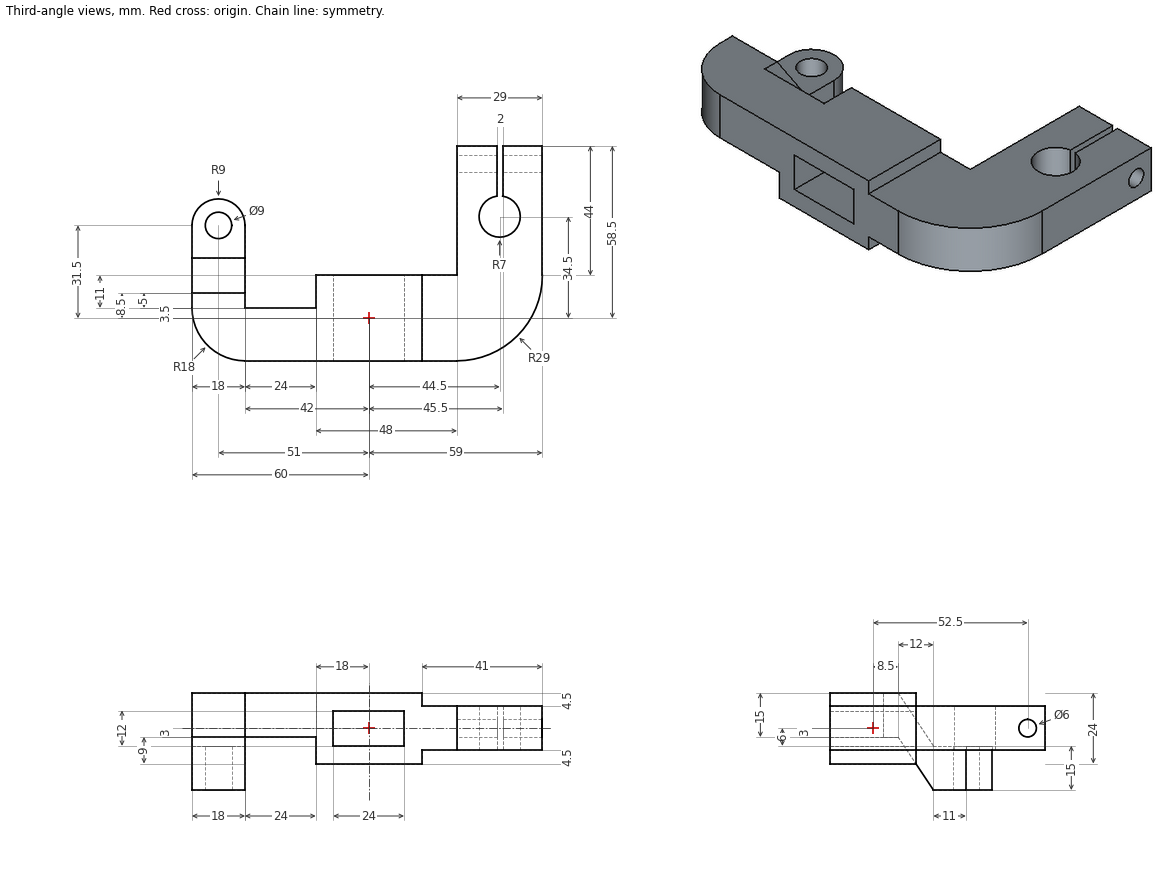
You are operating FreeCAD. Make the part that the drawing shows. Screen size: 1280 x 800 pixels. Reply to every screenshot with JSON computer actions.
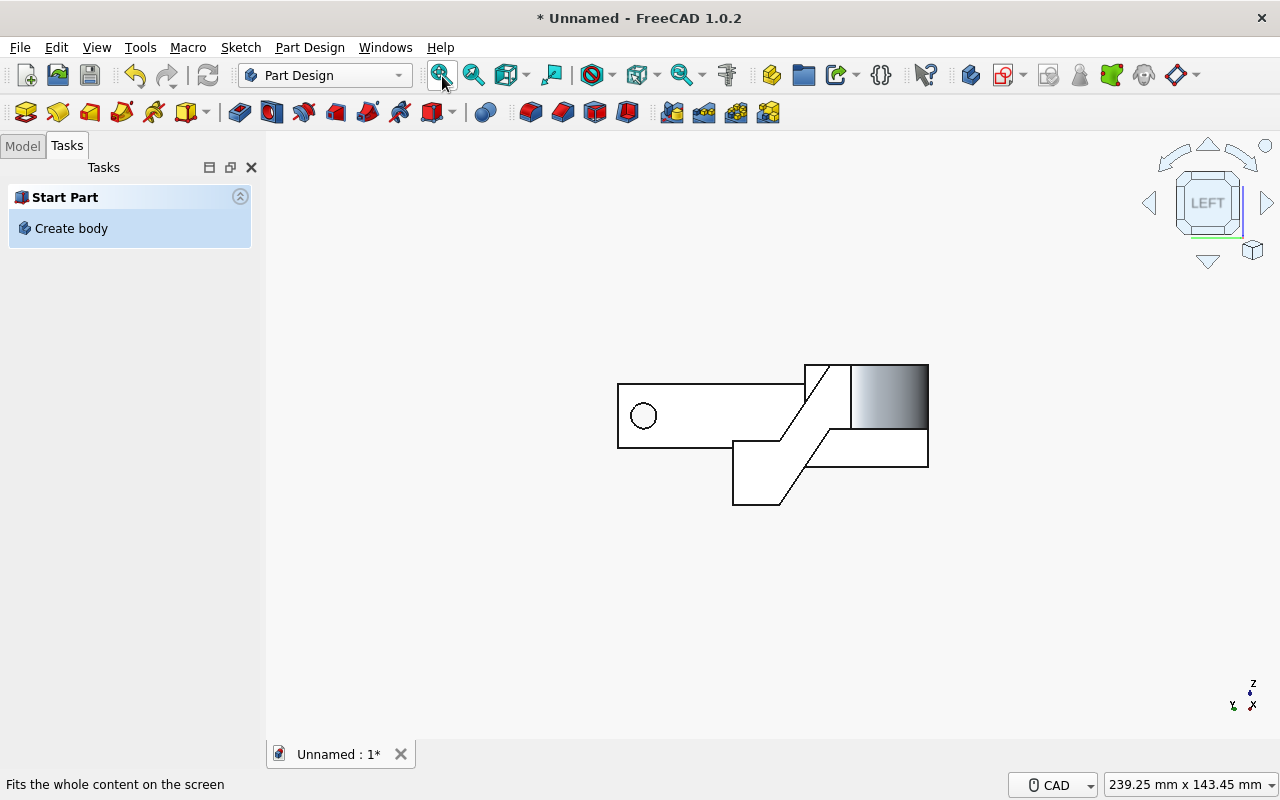
{"action": "key", "text": "0"}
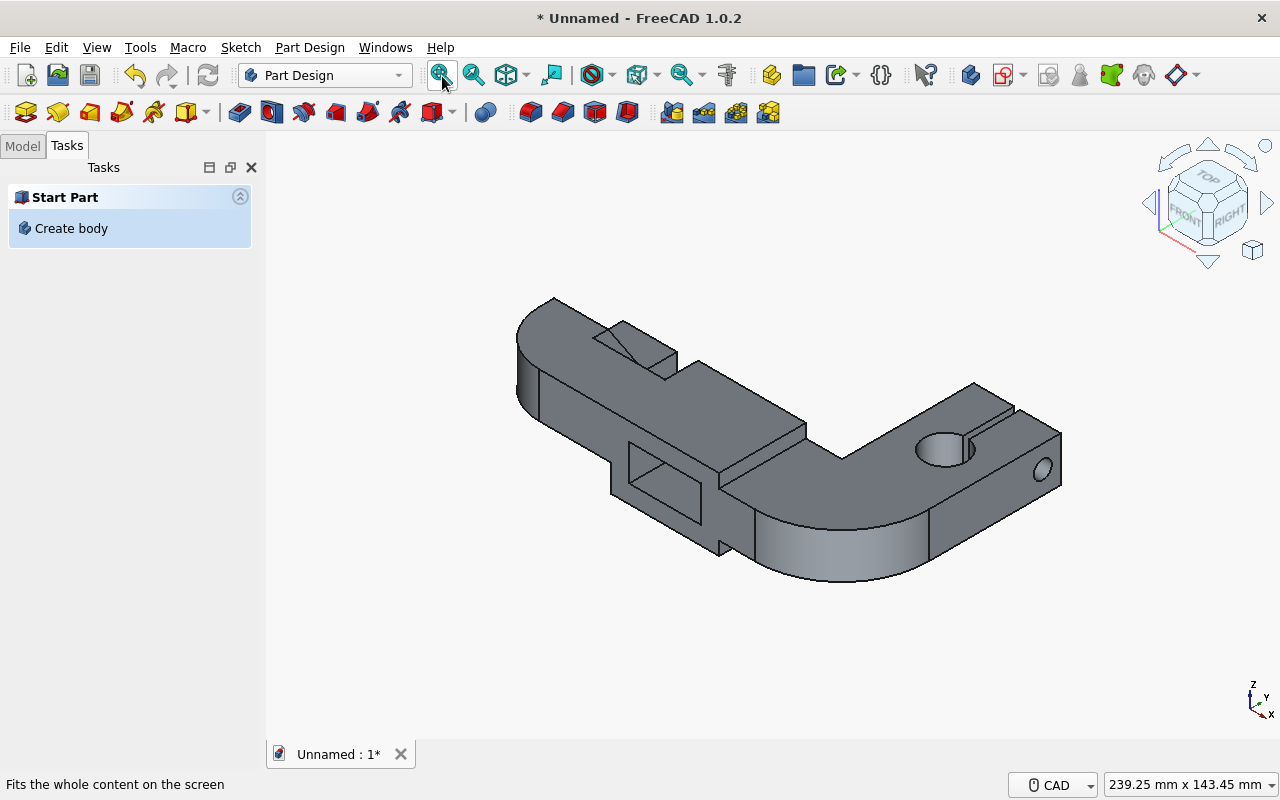
{"action": "left_click", "coordinate": [641, 349]}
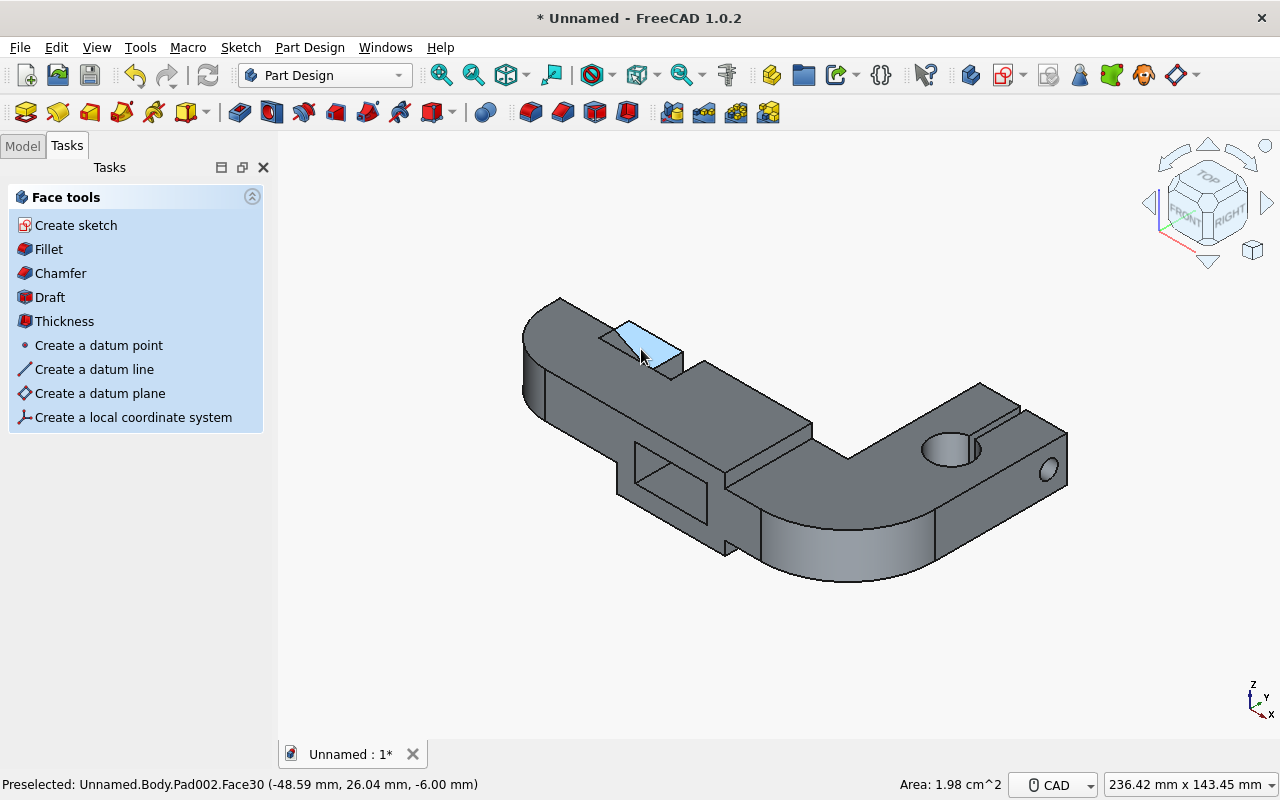
{"action": "left_click", "coordinate": [1004, 76]}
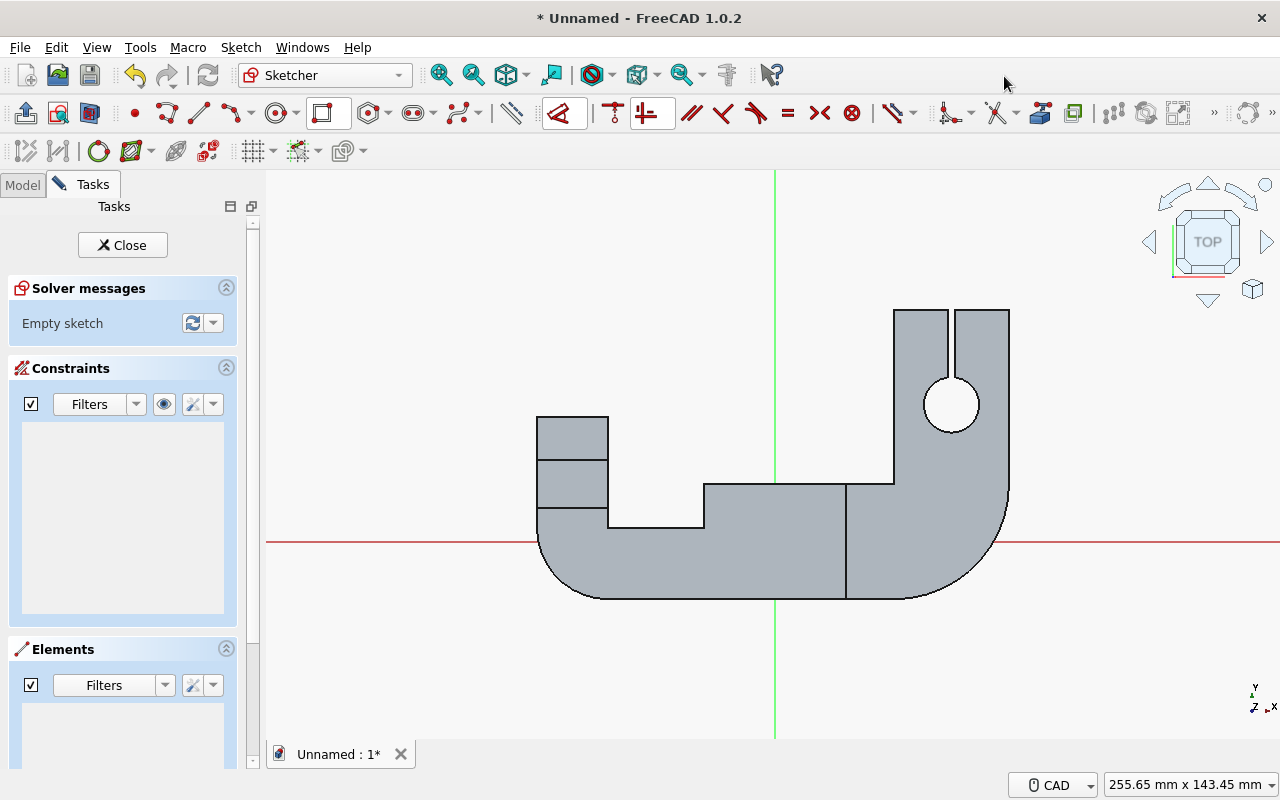
{"action": "scroll", "coordinate": [552, 390], "scroll_direction": "up", "scroll_amount": 10}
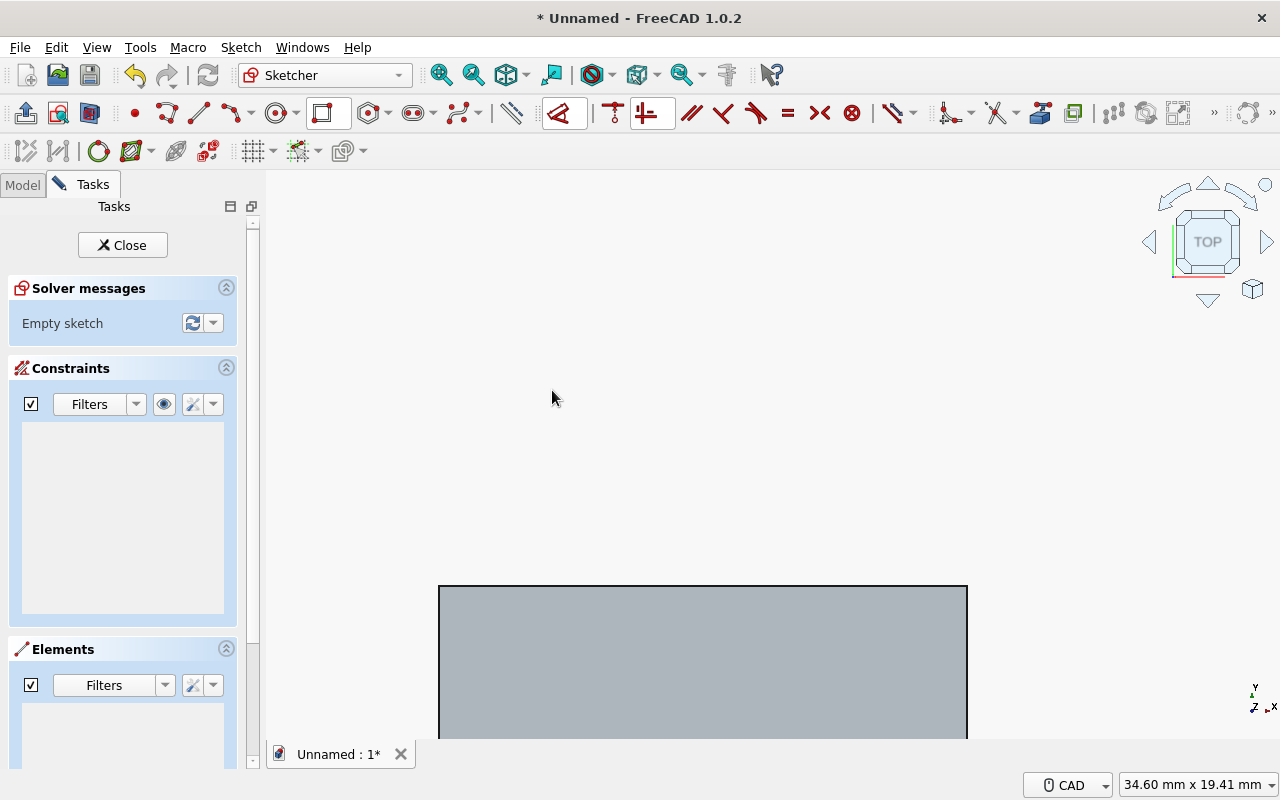
{"action": "left_click", "coordinate": [200, 114]}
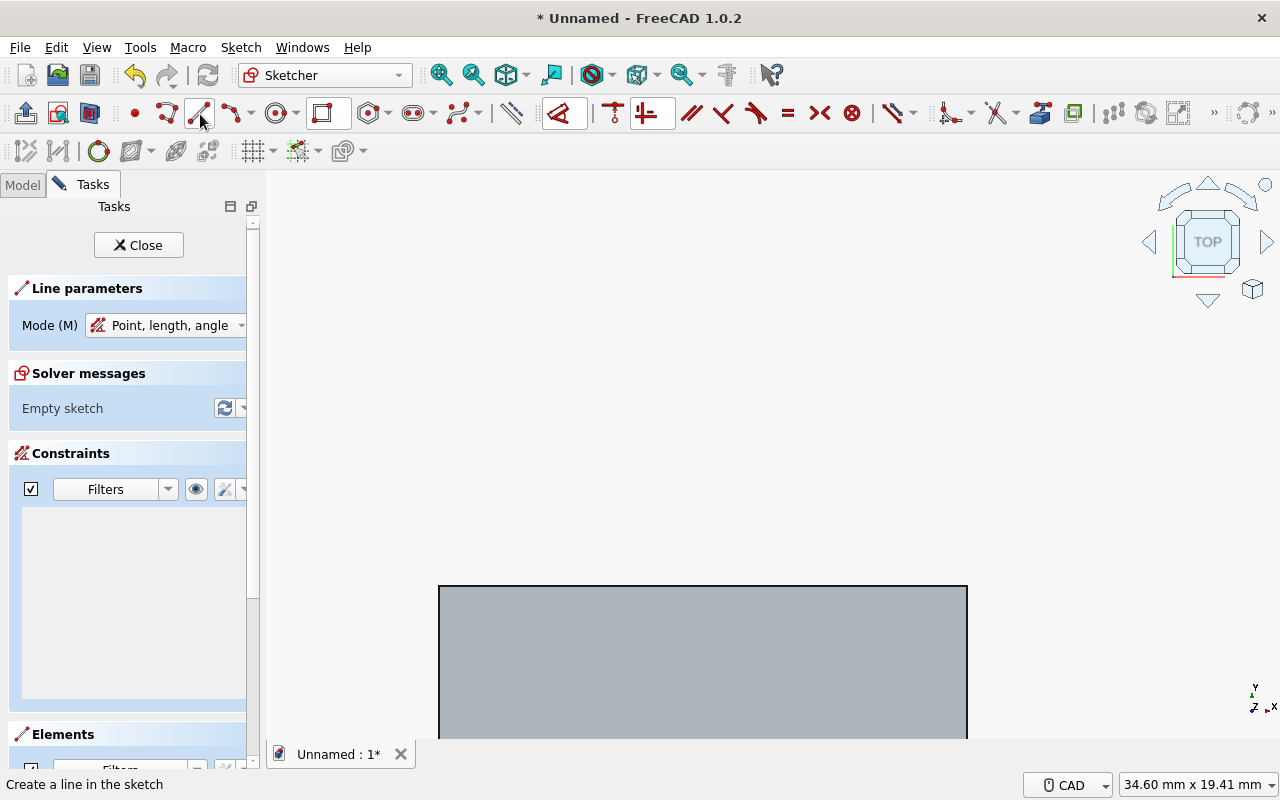
{"action": "left_click", "coordinate": [439, 586]}
{"action": "left_click", "coordinate": [967, 586]}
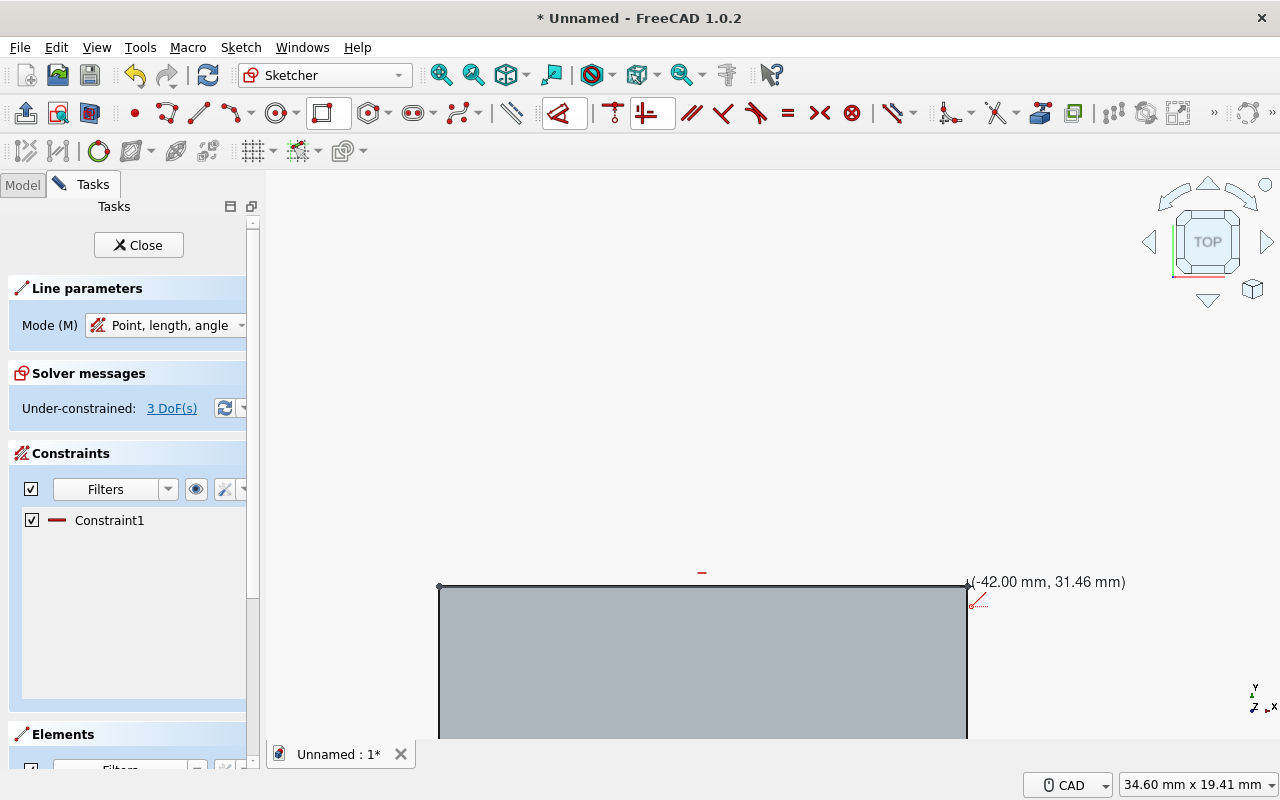
{"action": "left_click", "coordinate": [232, 114]}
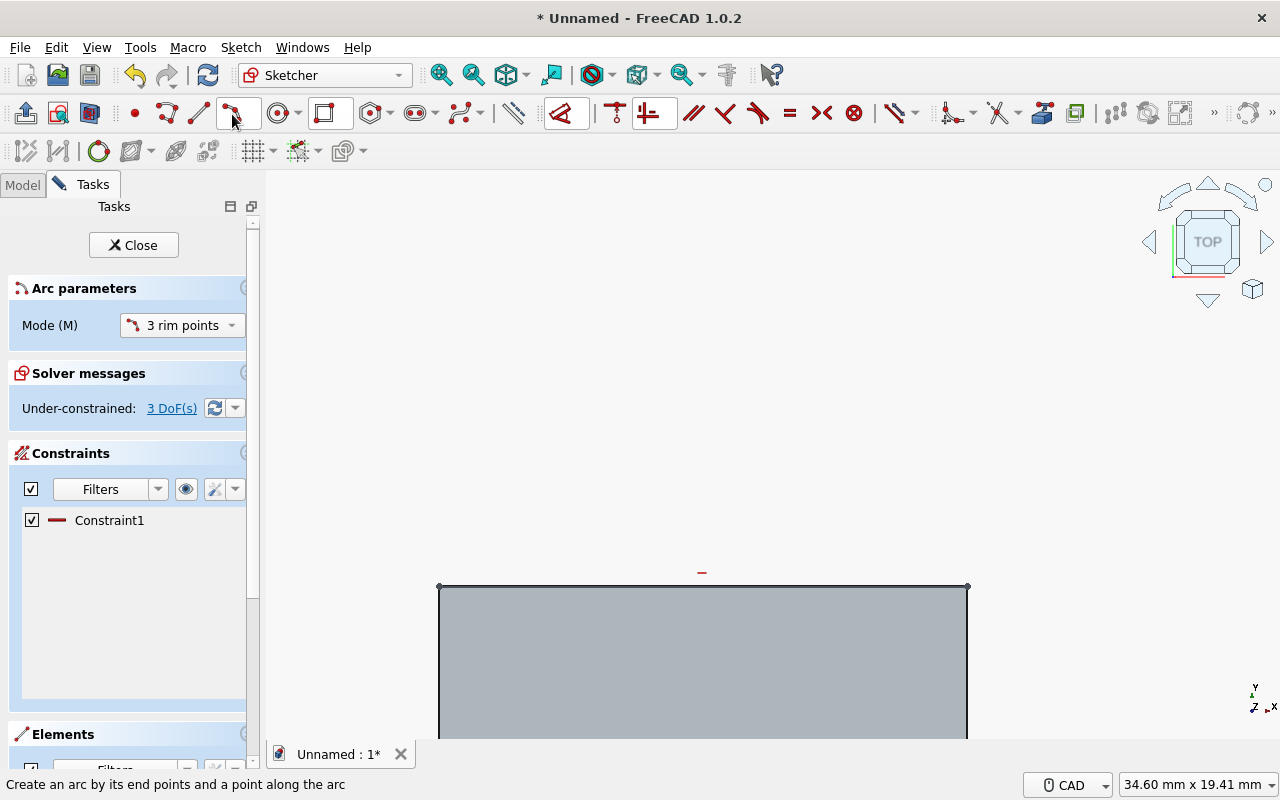
{"action": "left_click", "coordinate": [967, 587]}
{"action": "left_click", "coordinate": [439, 587]}
{"action": "left_click", "coordinate": [703, 322]}
{"action": "key", "text": "Escape"}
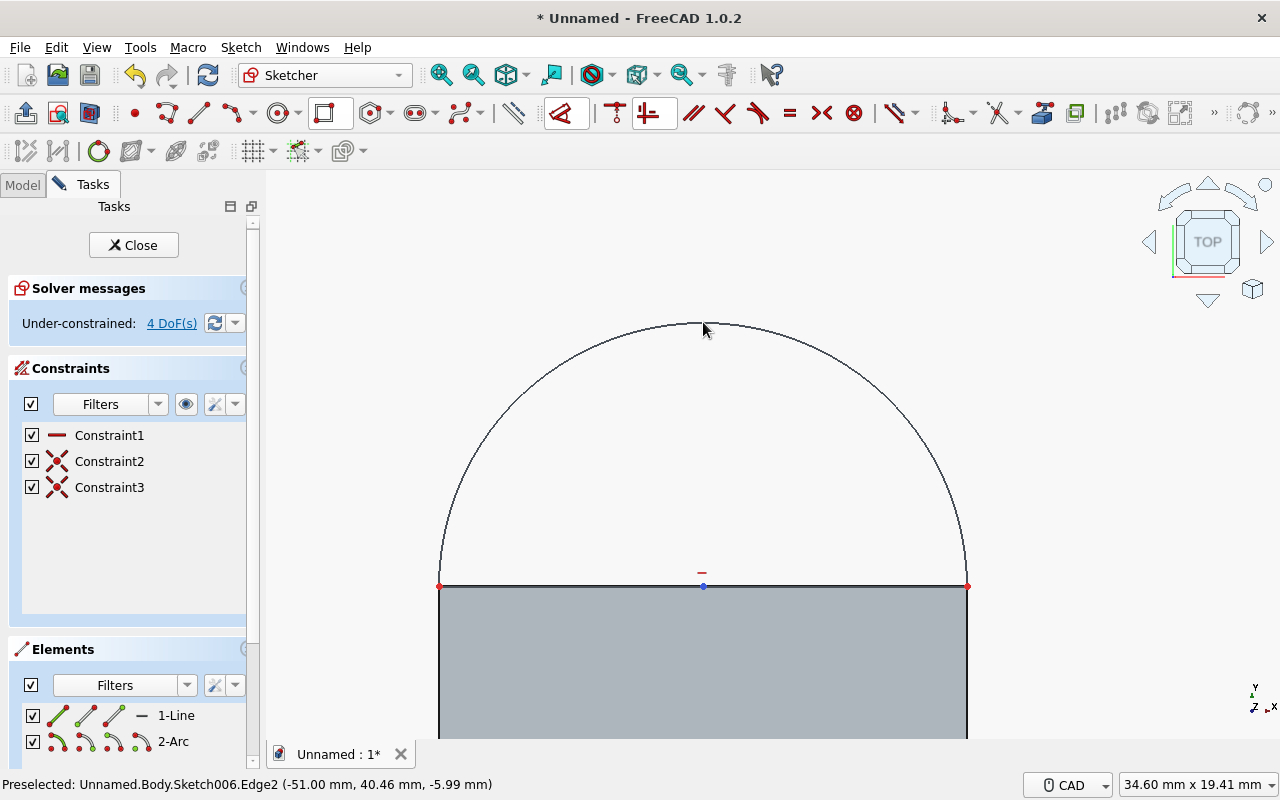
{"action": "left_click", "coordinate": [858, 373]}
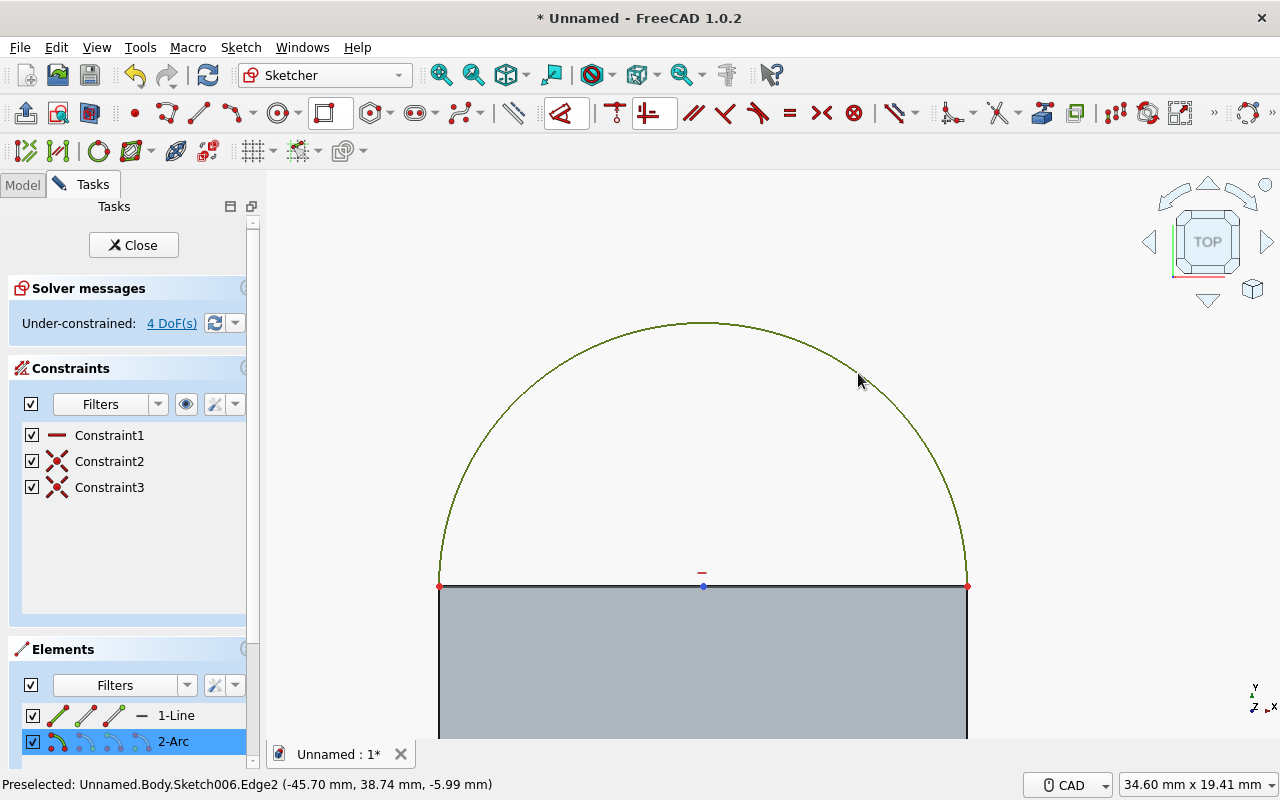
{"action": "key", "text": "k r"}